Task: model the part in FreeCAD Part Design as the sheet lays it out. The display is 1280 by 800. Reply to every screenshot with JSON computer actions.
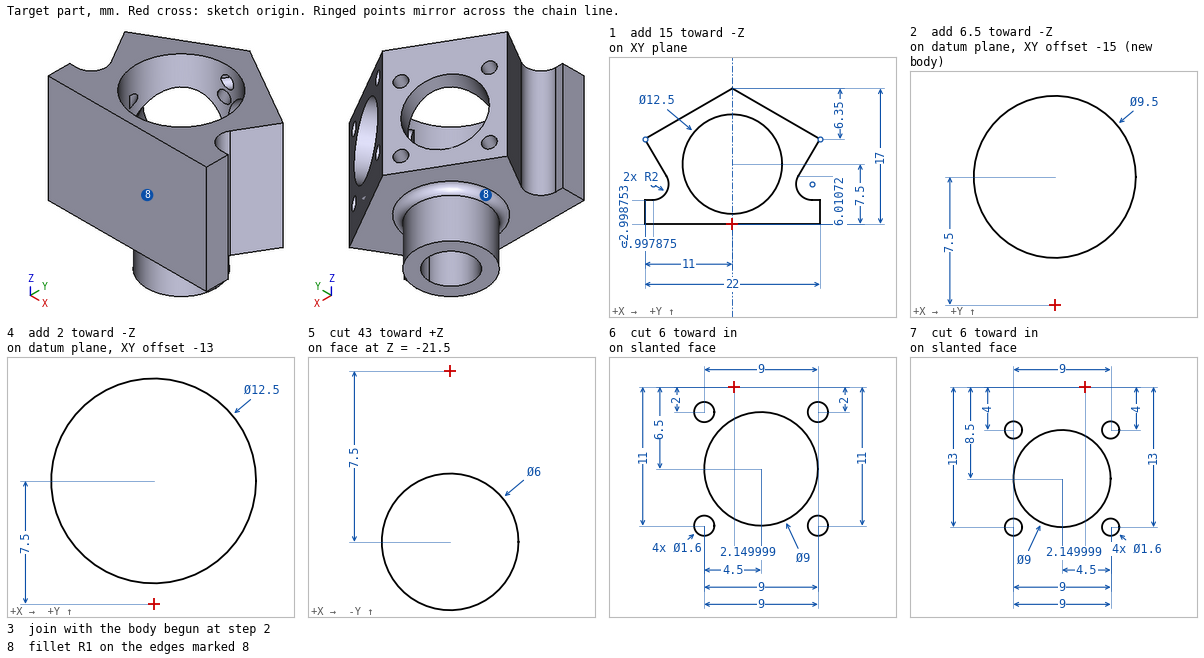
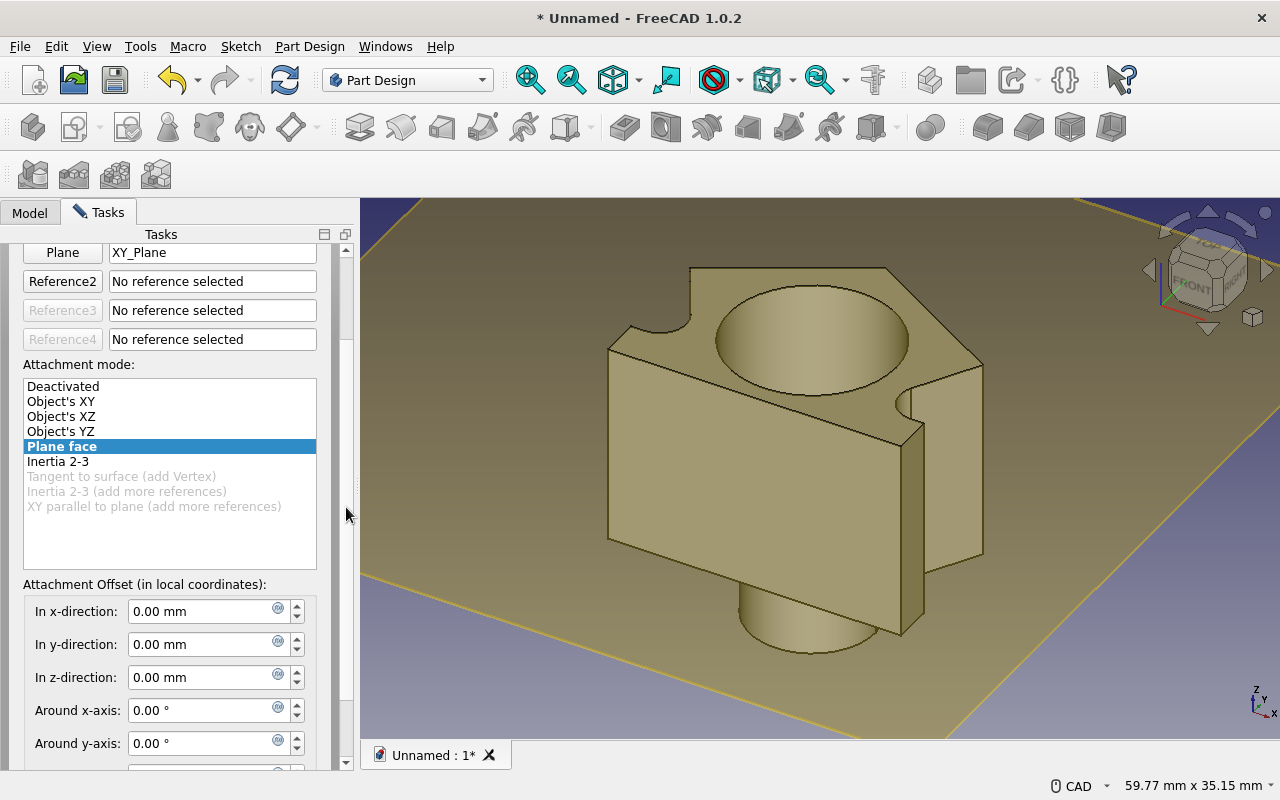
{"action": "triple_click", "coordinate": [210, 678]}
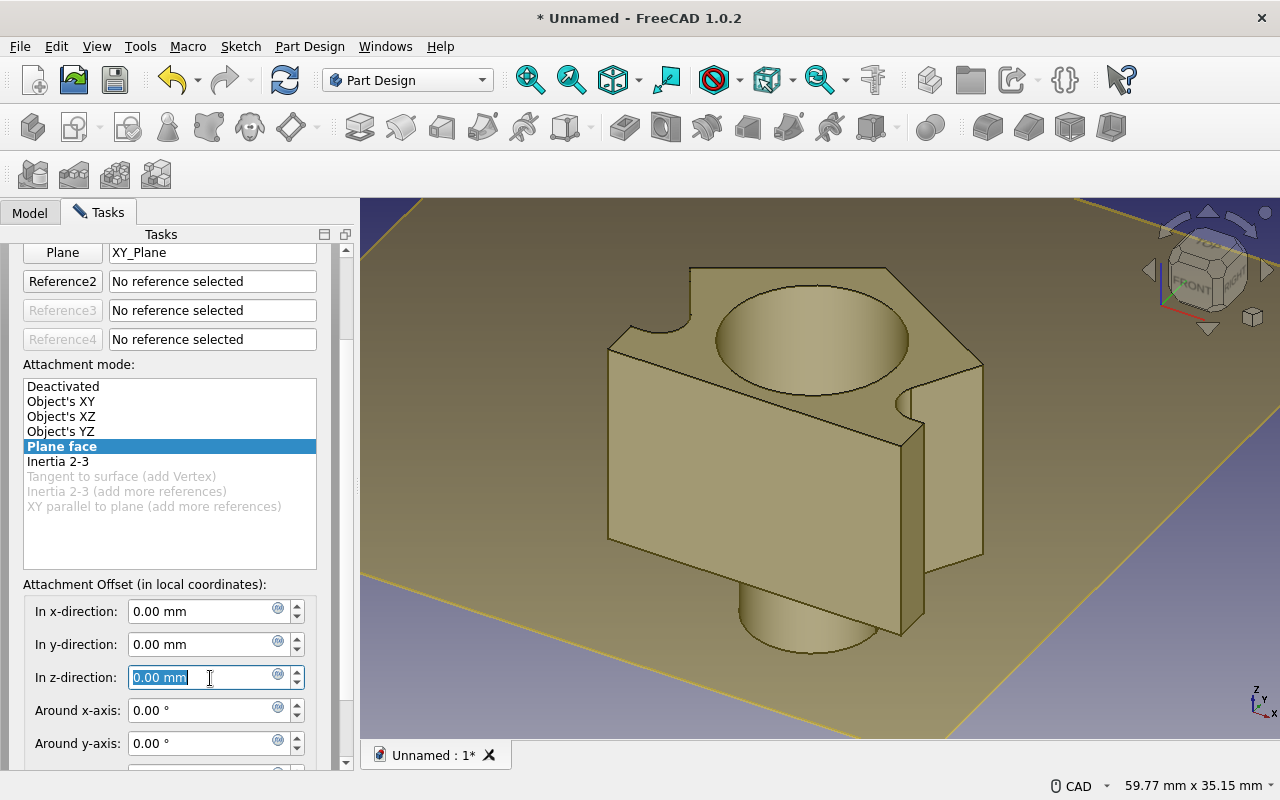
{"action": "type", "text": "-13"}
{"action": "key", "text": "Tab"}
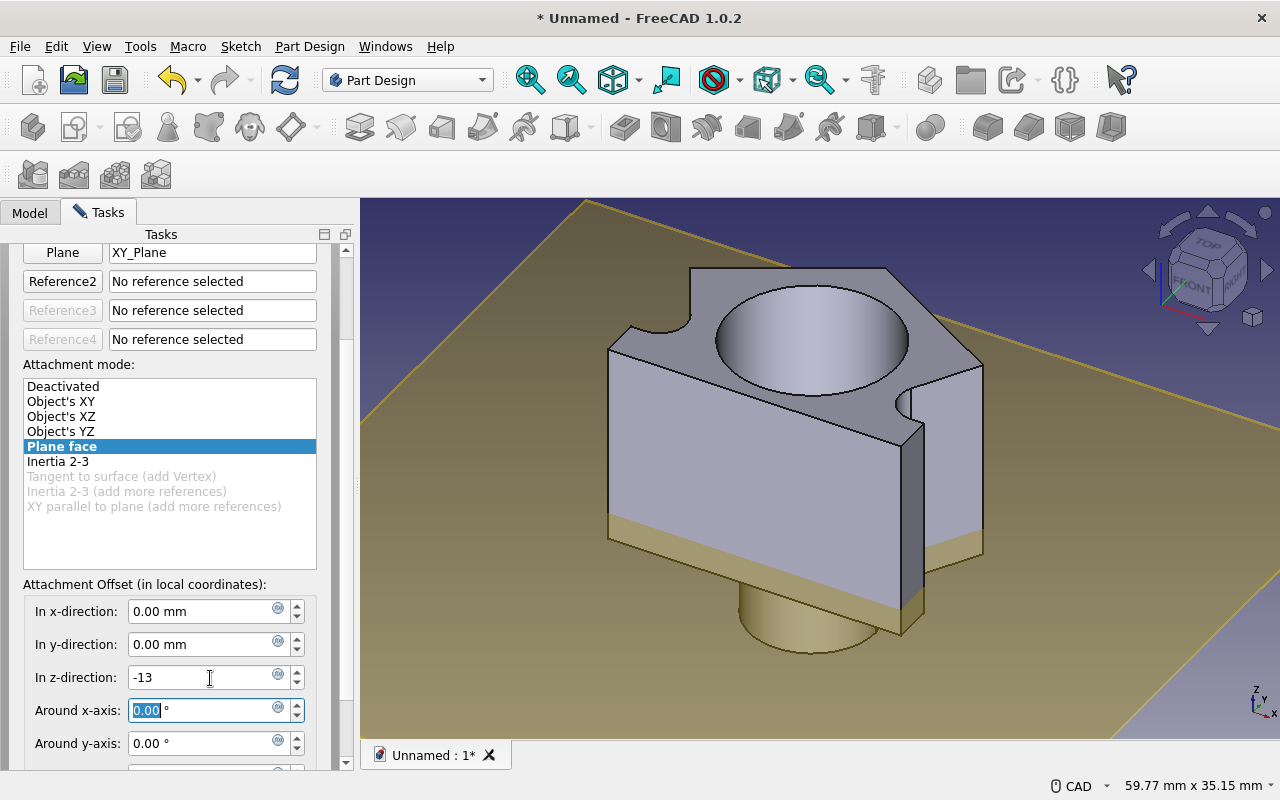
{"action": "scroll", "coordinate": [346, 507], "scroll_direction": "up", "scroll_amount": 3}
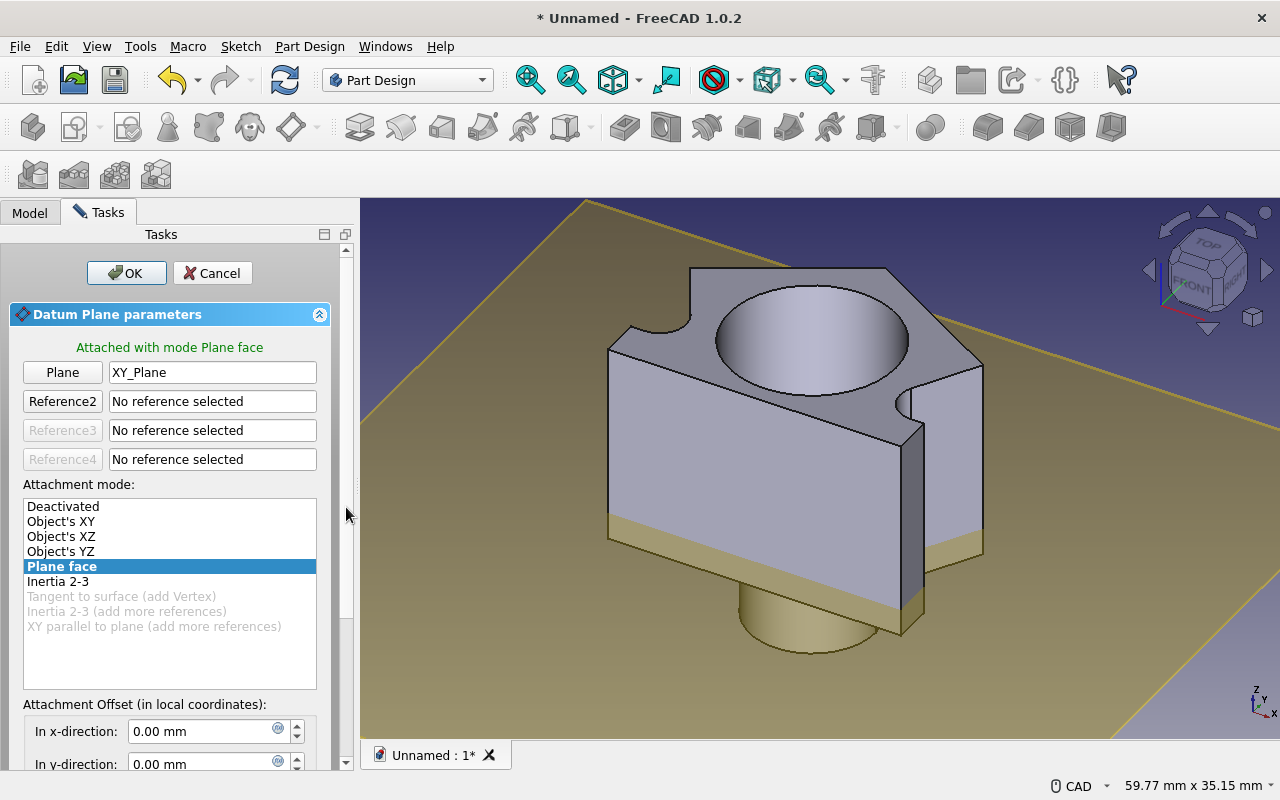
{"action": "left_click", "coordinate": [127, 273]}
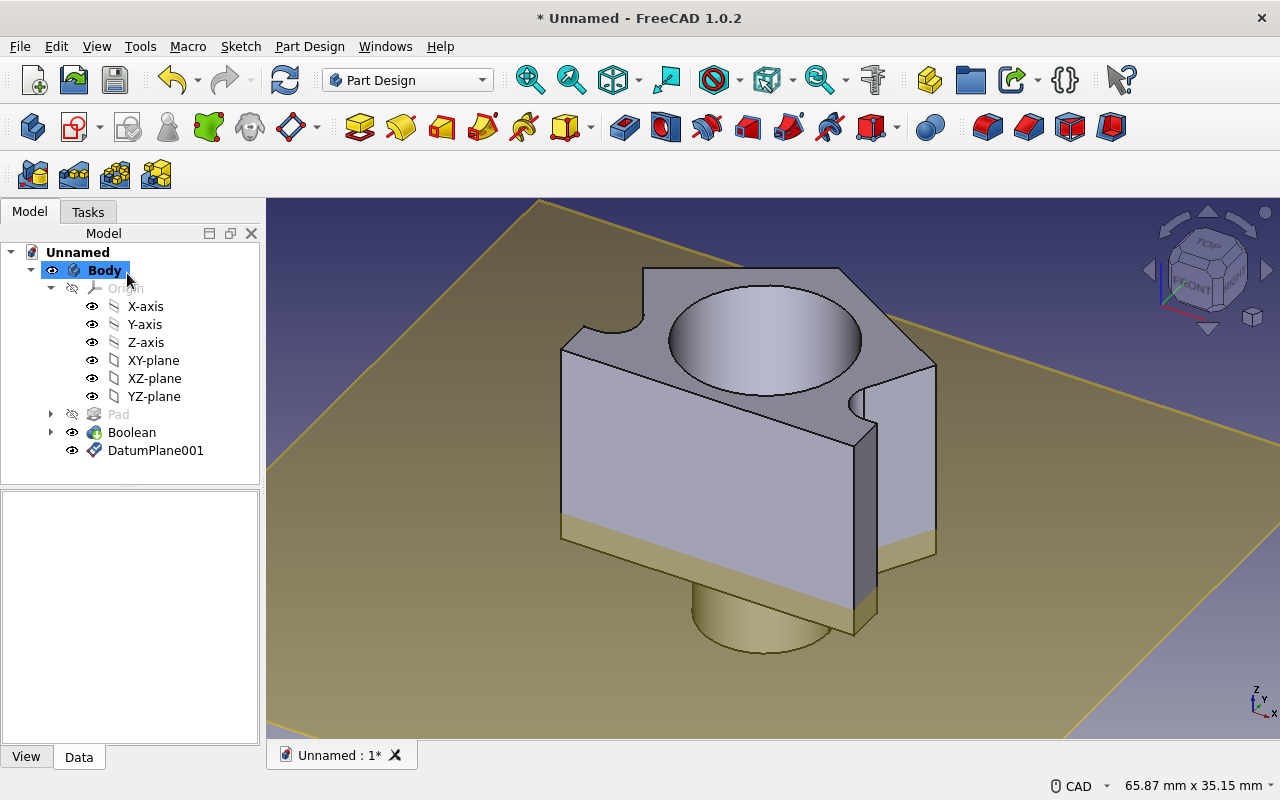
{"action": "left_click", "coordinate": [117, 450]}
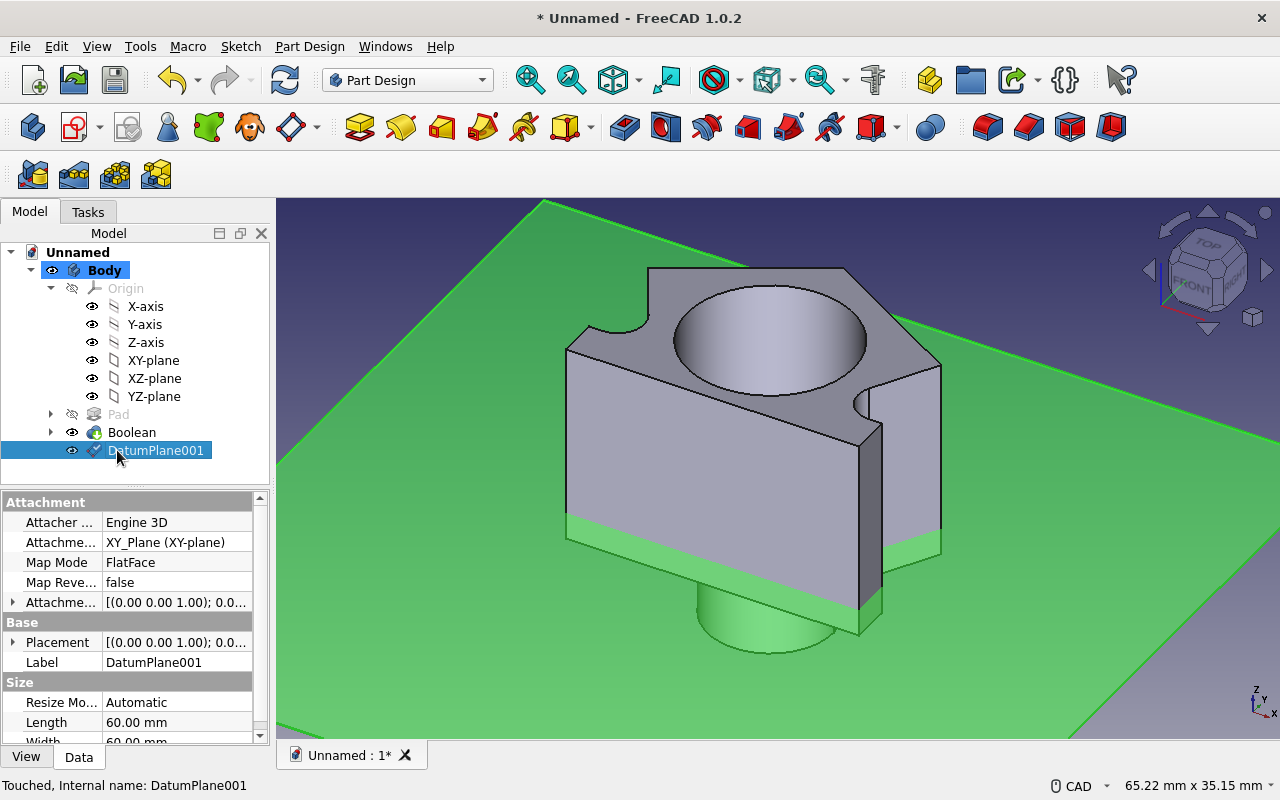
{"action": "left_click", "coordinate": [74, 128]}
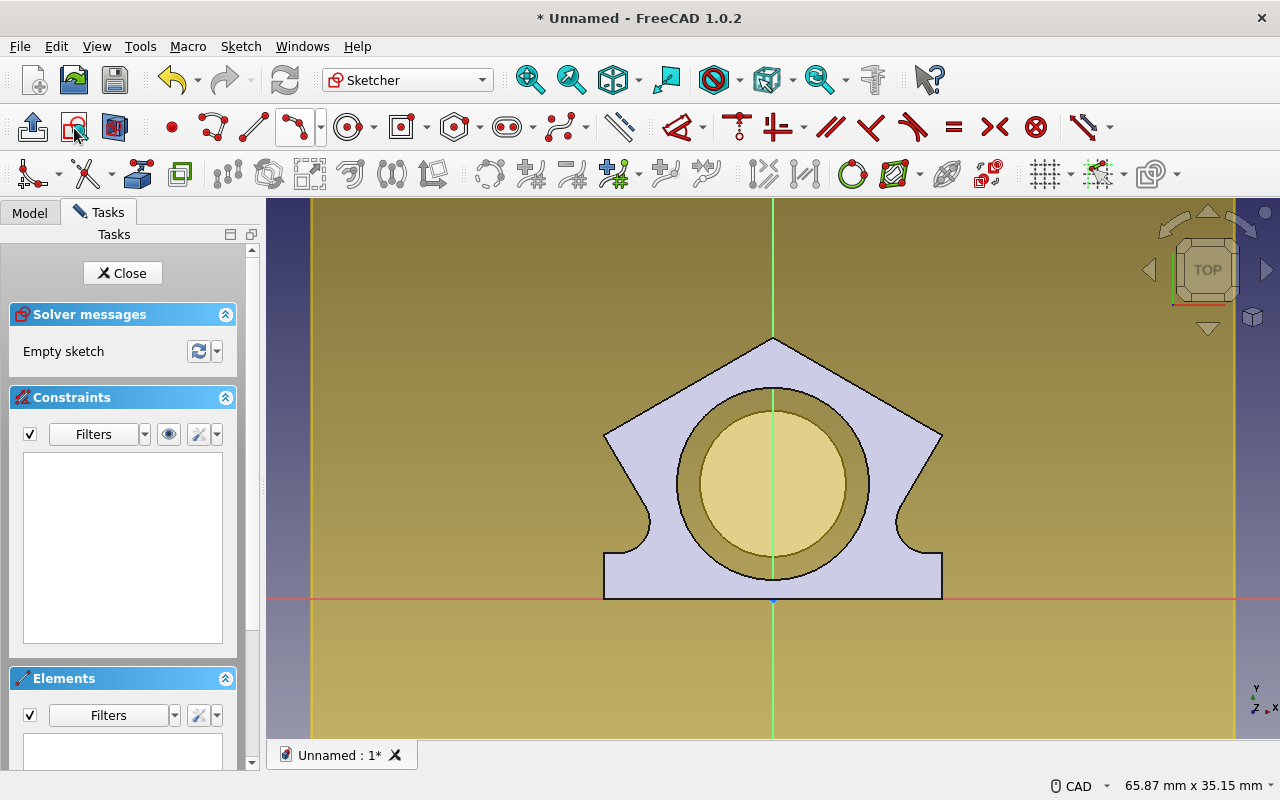
{"action": "left_click", "coordinate": [115, 128]}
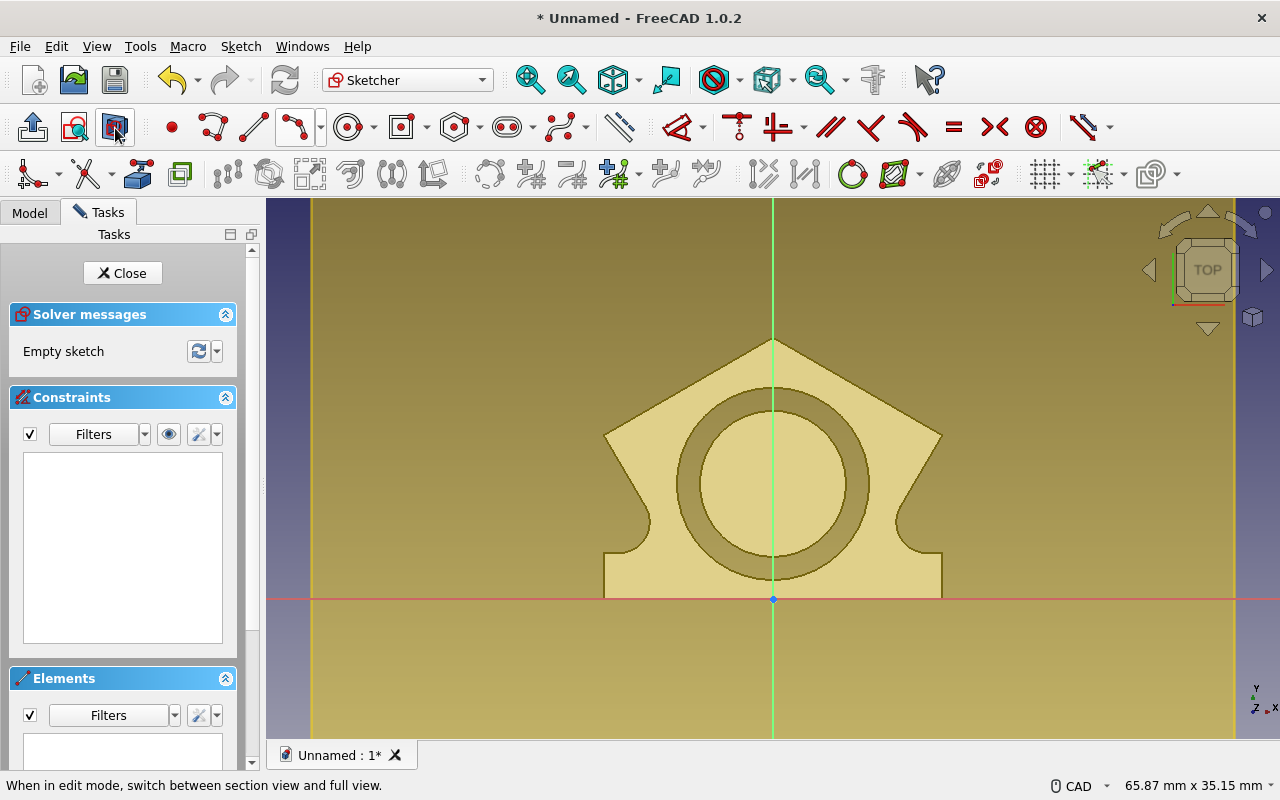
{"action": "scroll", "coordinate": [912, 544], "scroll_direction": "up", "scroll_amount": 2}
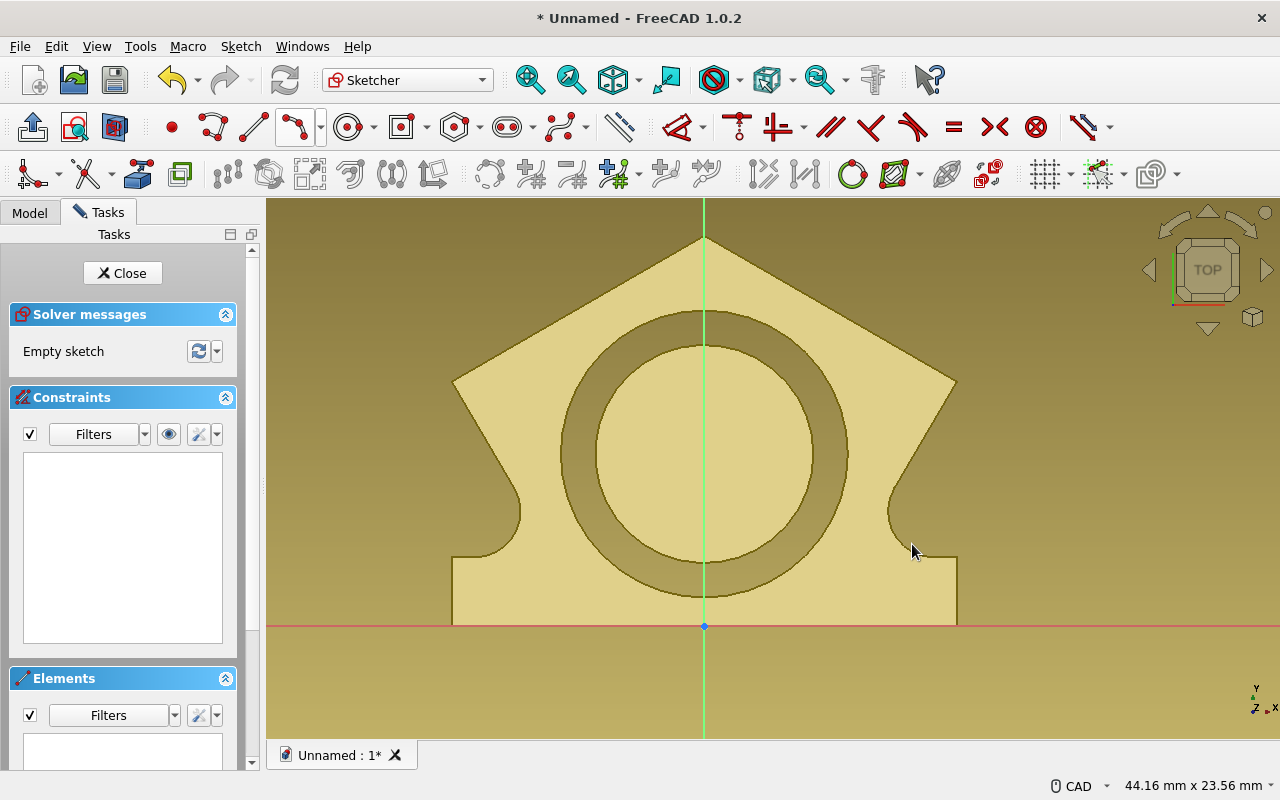
{"action": "left_click", "coordinate": [348, 128]}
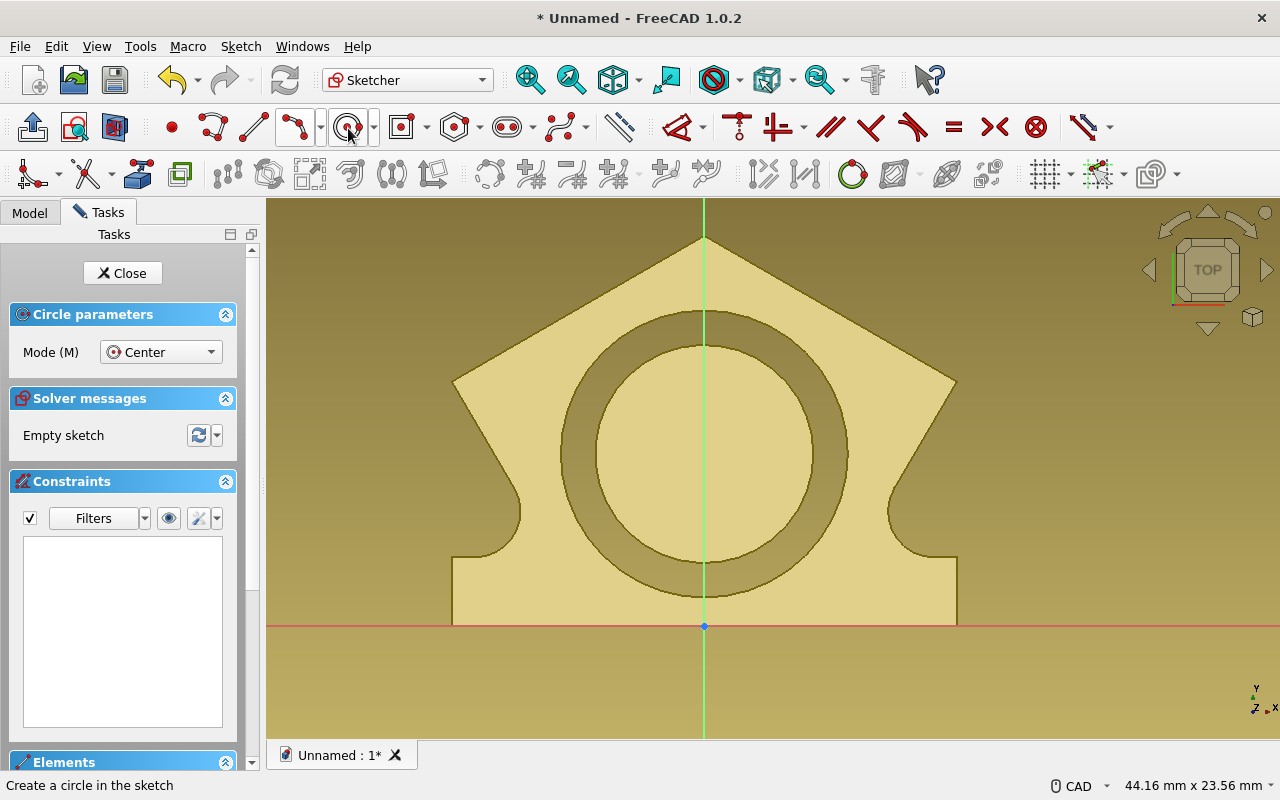
{"action": "left_click", "coordinate": [704, 454]}
{"action": "mouse_move", "coordinate": [806, 353]}